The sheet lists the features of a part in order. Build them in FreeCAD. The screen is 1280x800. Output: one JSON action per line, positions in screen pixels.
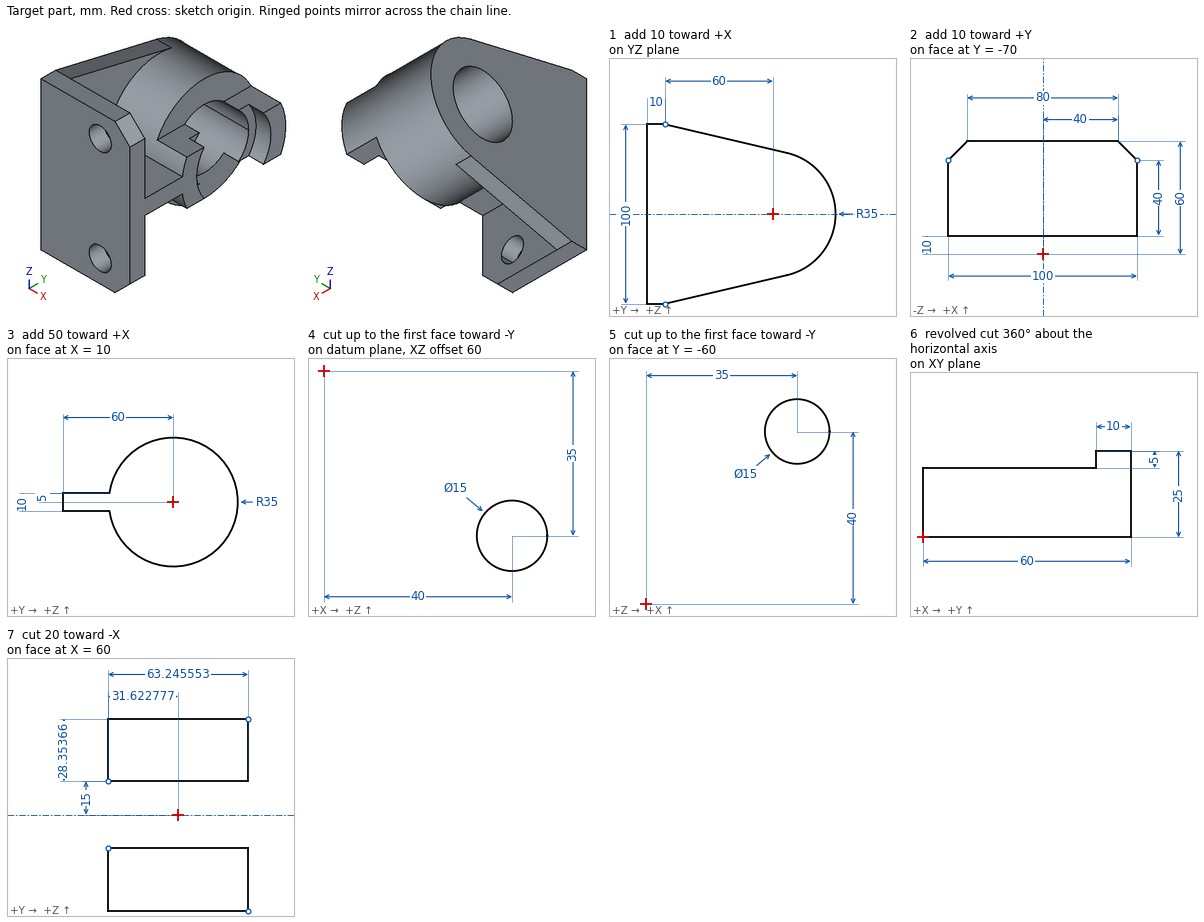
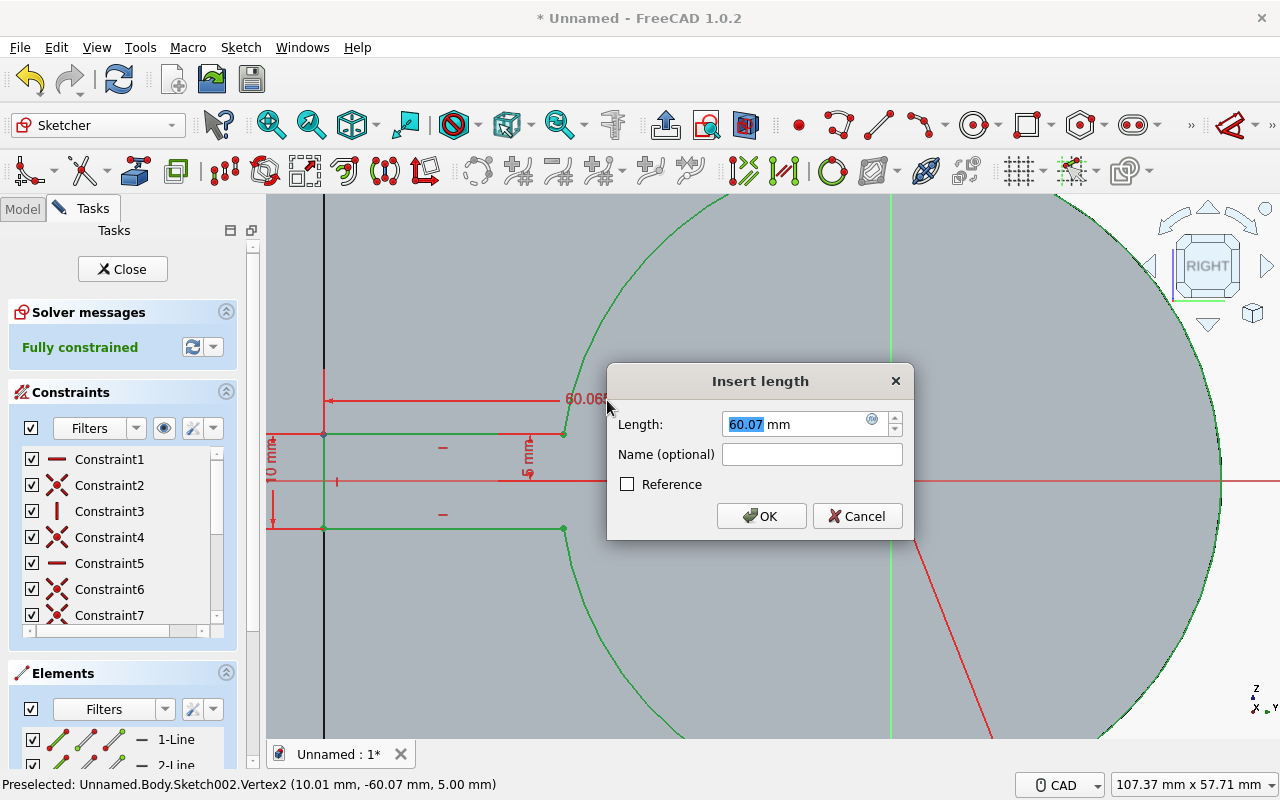
{"action": "type", "text": "60"}
{"action": "key", "text": "Return"}
{"action": "key", "text": "Escape"}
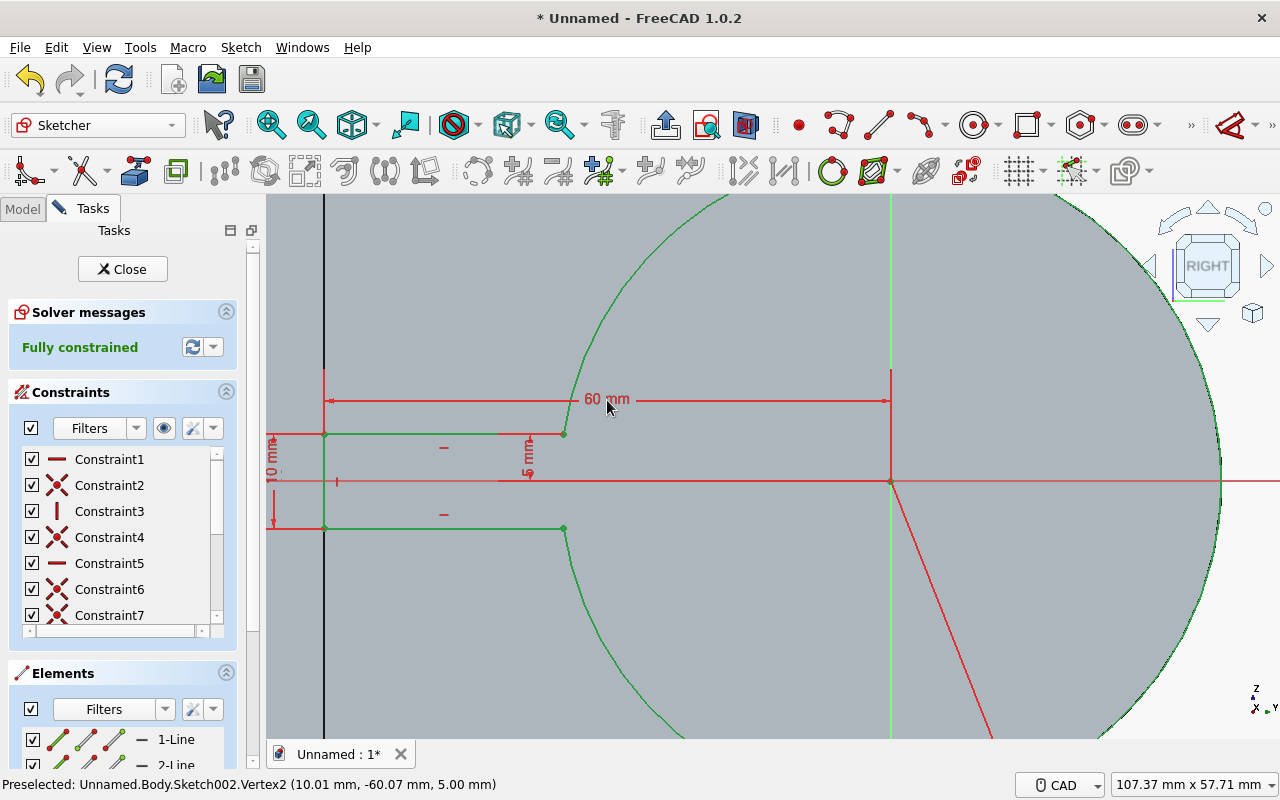
{"action": "left_click", "coordinate": [123, 269]}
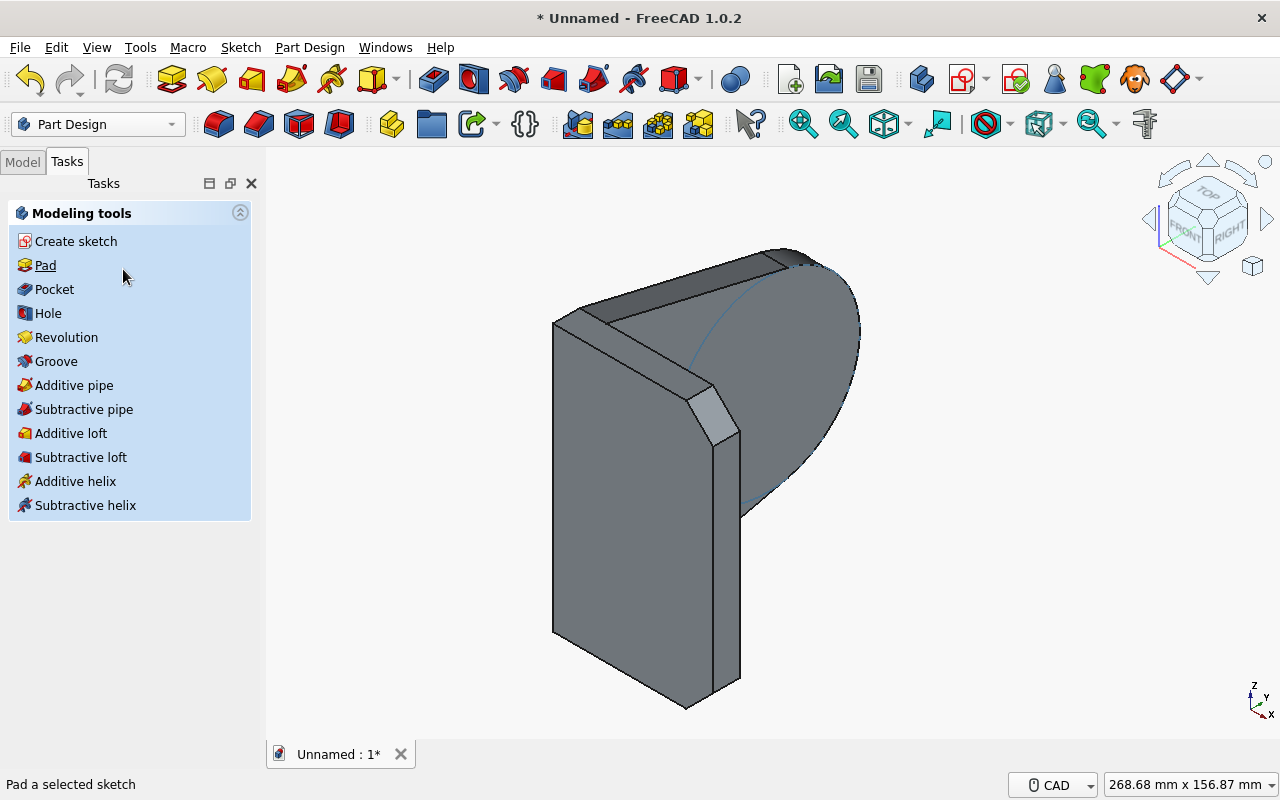
{"action": "left_click", "coordinate": [172, 80]}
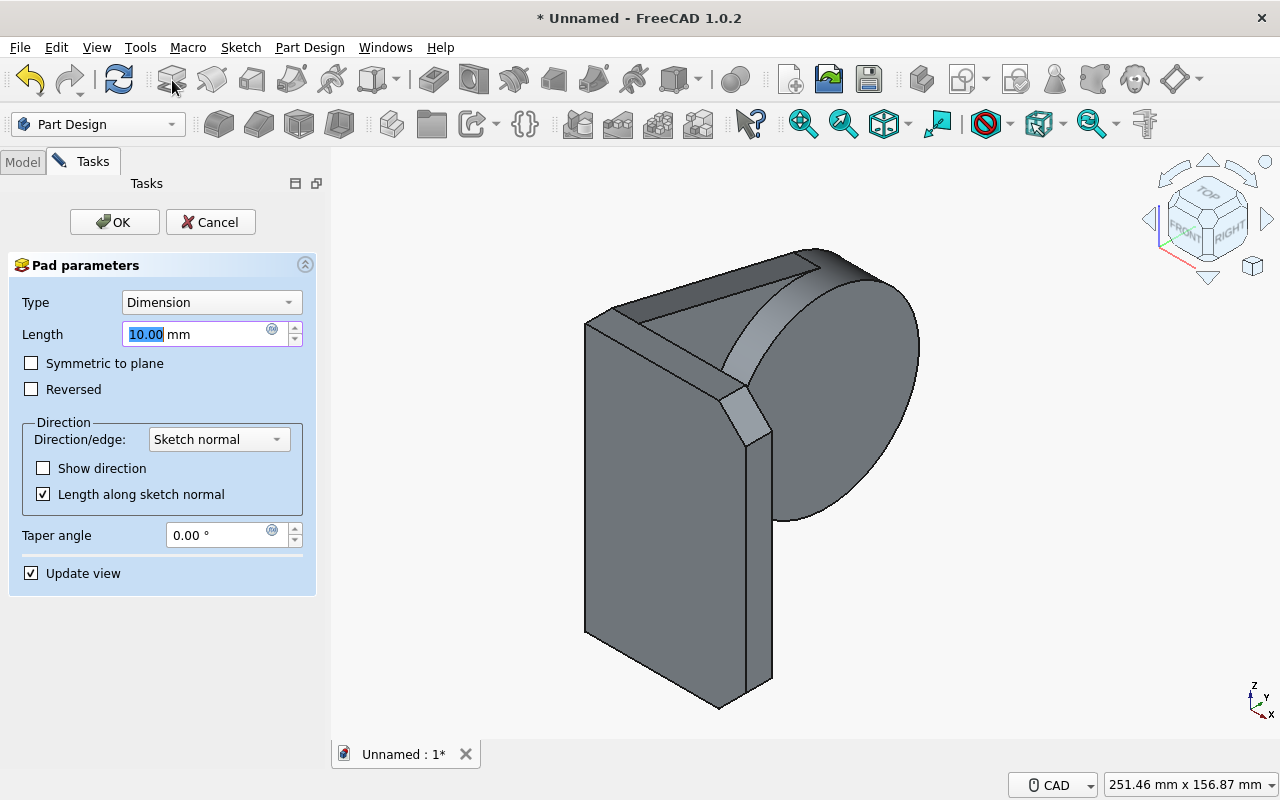
{"action": "type", "text": "50"}
{"action": "key", "text": "Tab"}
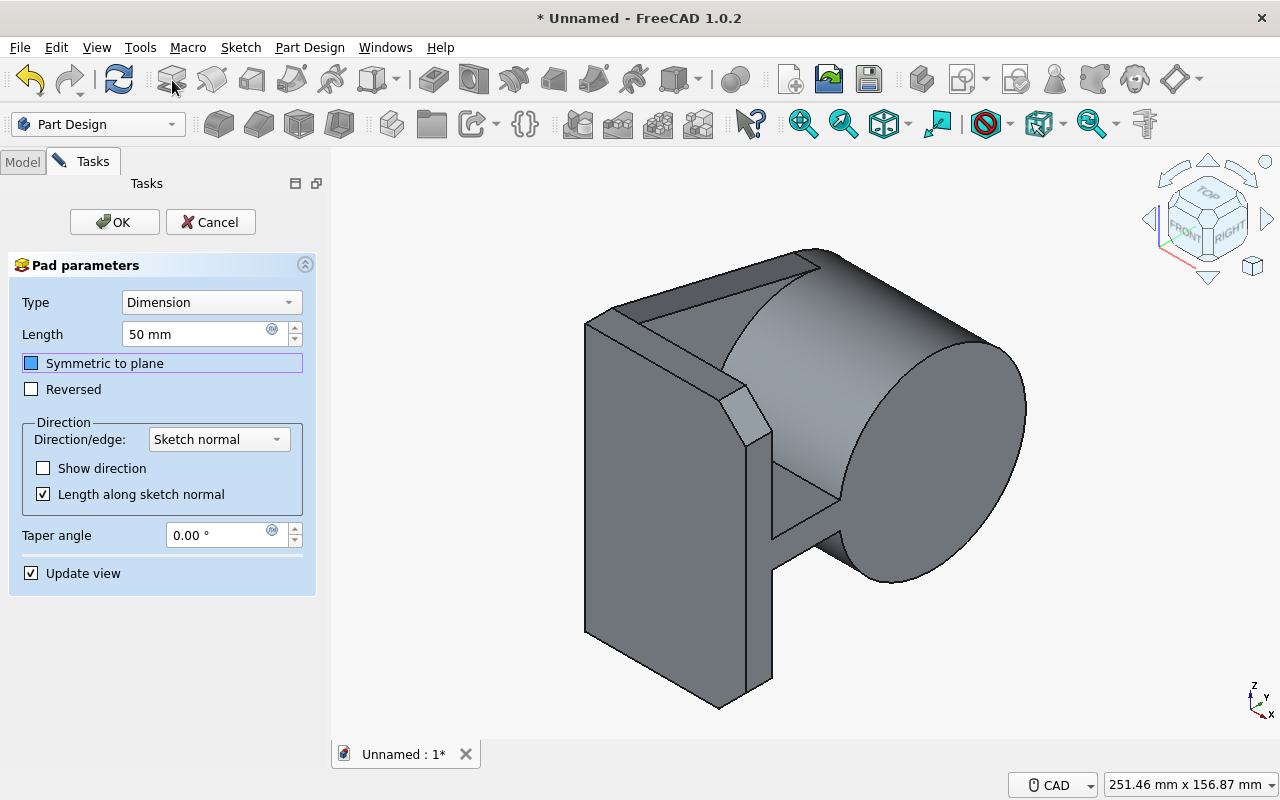
{"action": "left_click", "coordinate": [115, 222]}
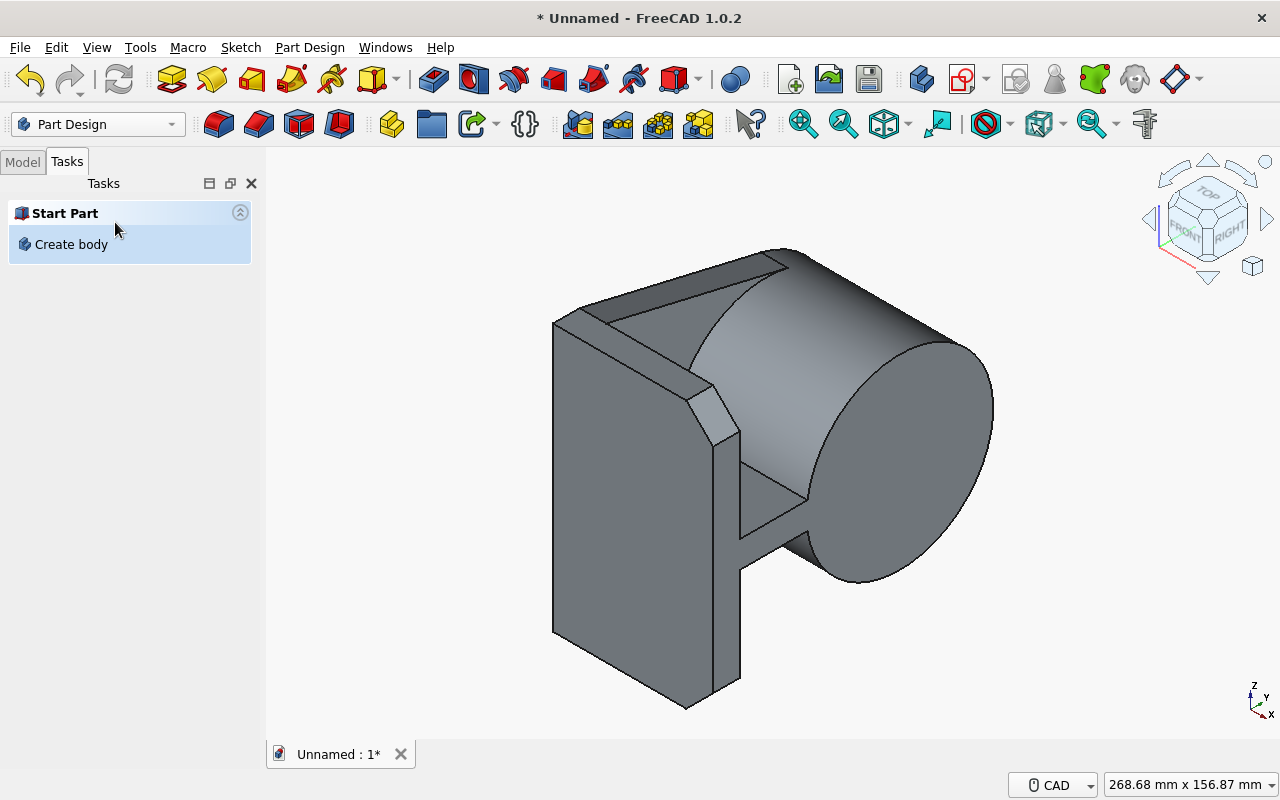
{"action": "left_click", "coordinate": [23, 161]}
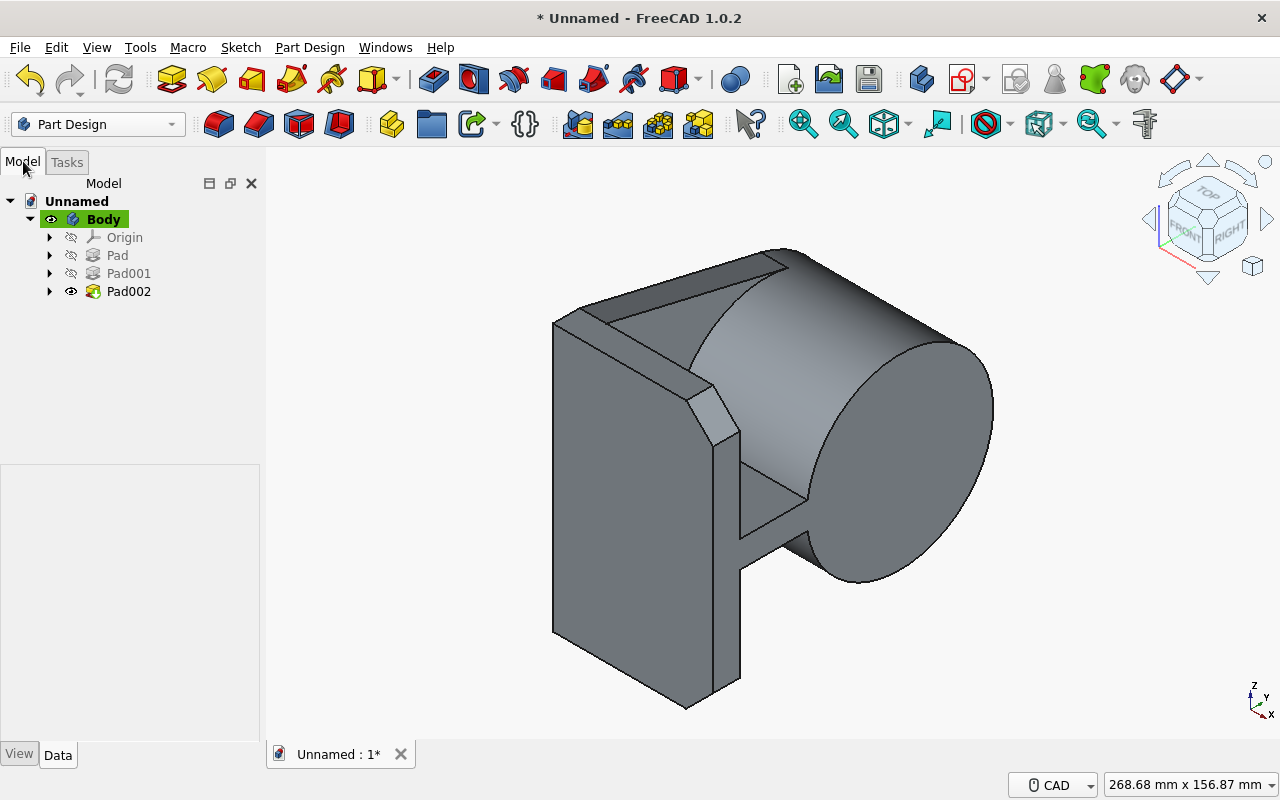
{"action": "left_click", "coordinate": [50, 237]}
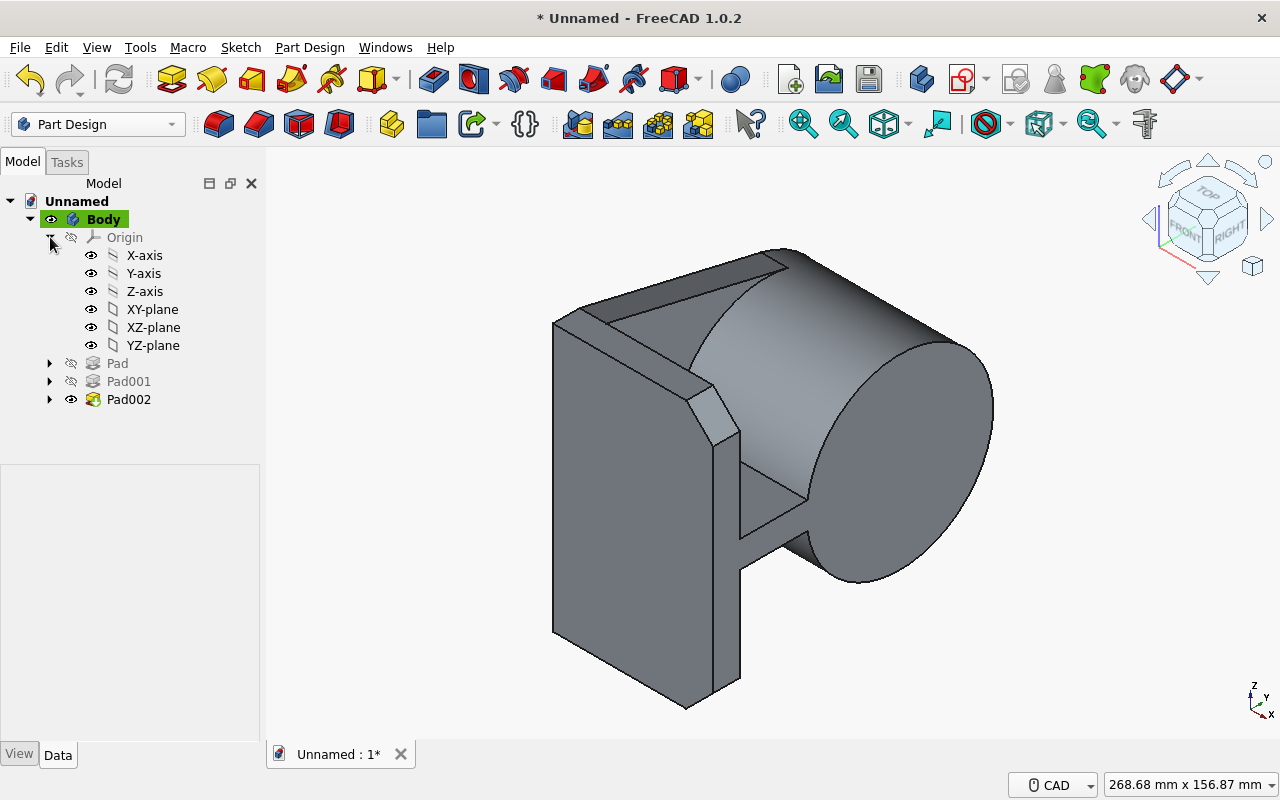
{"action": "left_click", "coordinate": [136, 327]}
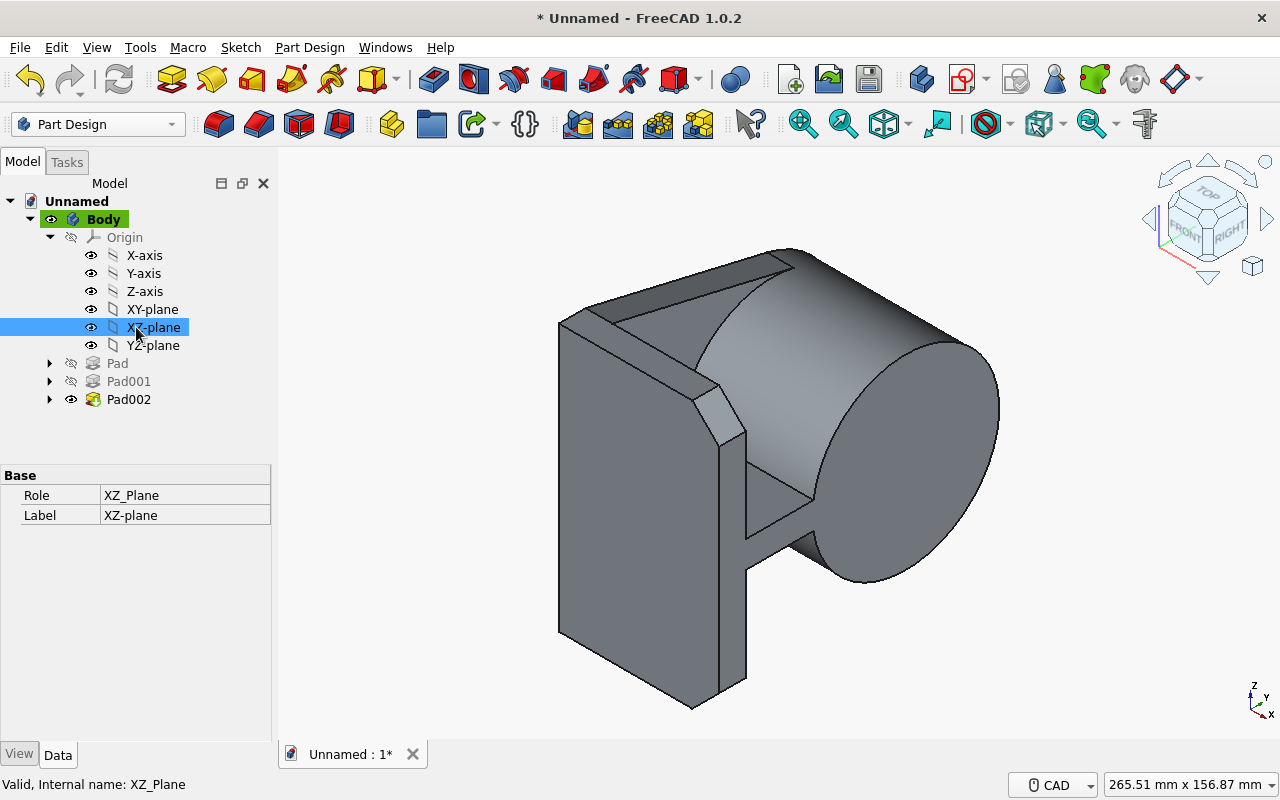
{"action": "left_click", "coordinate": [1176, 80]}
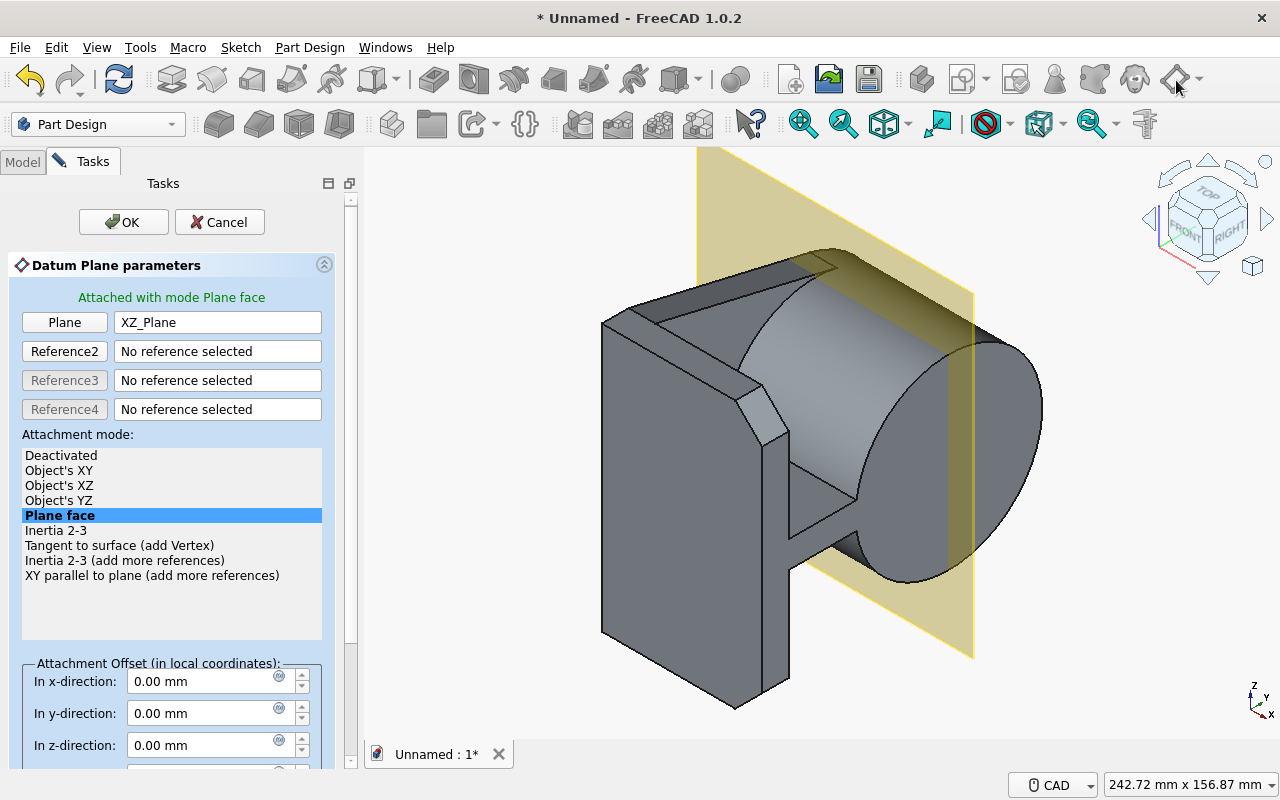
{"action": "triple_click", "coordinate": [210, 745]}